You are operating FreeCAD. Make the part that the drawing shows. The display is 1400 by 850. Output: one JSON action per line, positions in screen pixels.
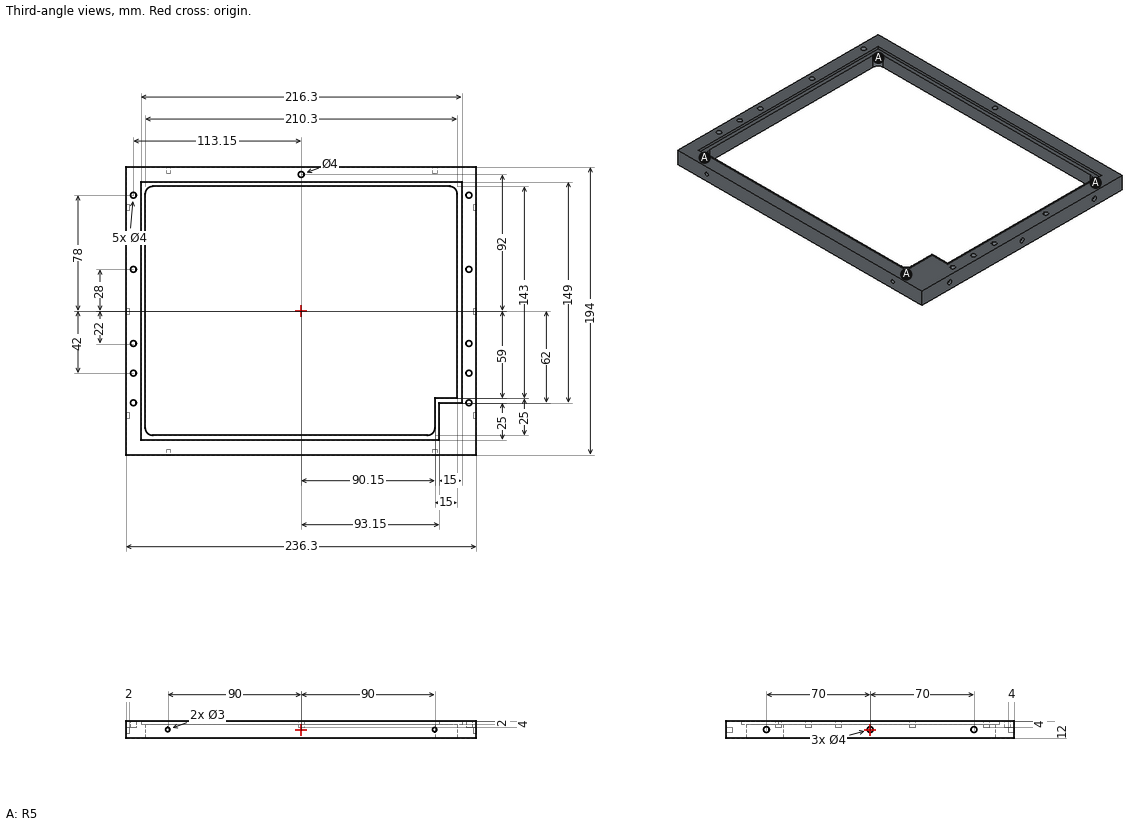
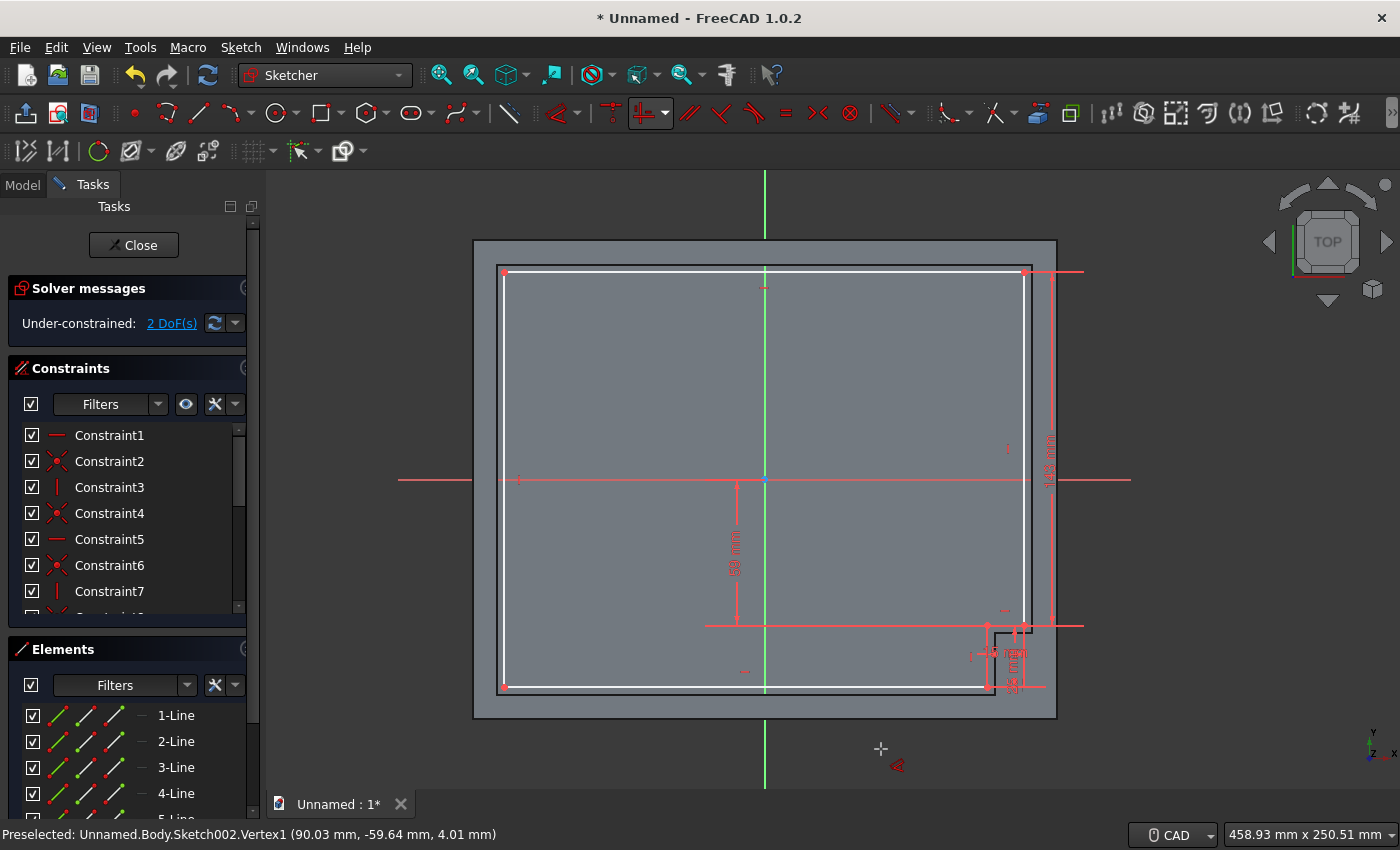
{"action": "left_click", "coordinate": [868, 272]}
{"action": "left_click", "coordinate": [645, 238]}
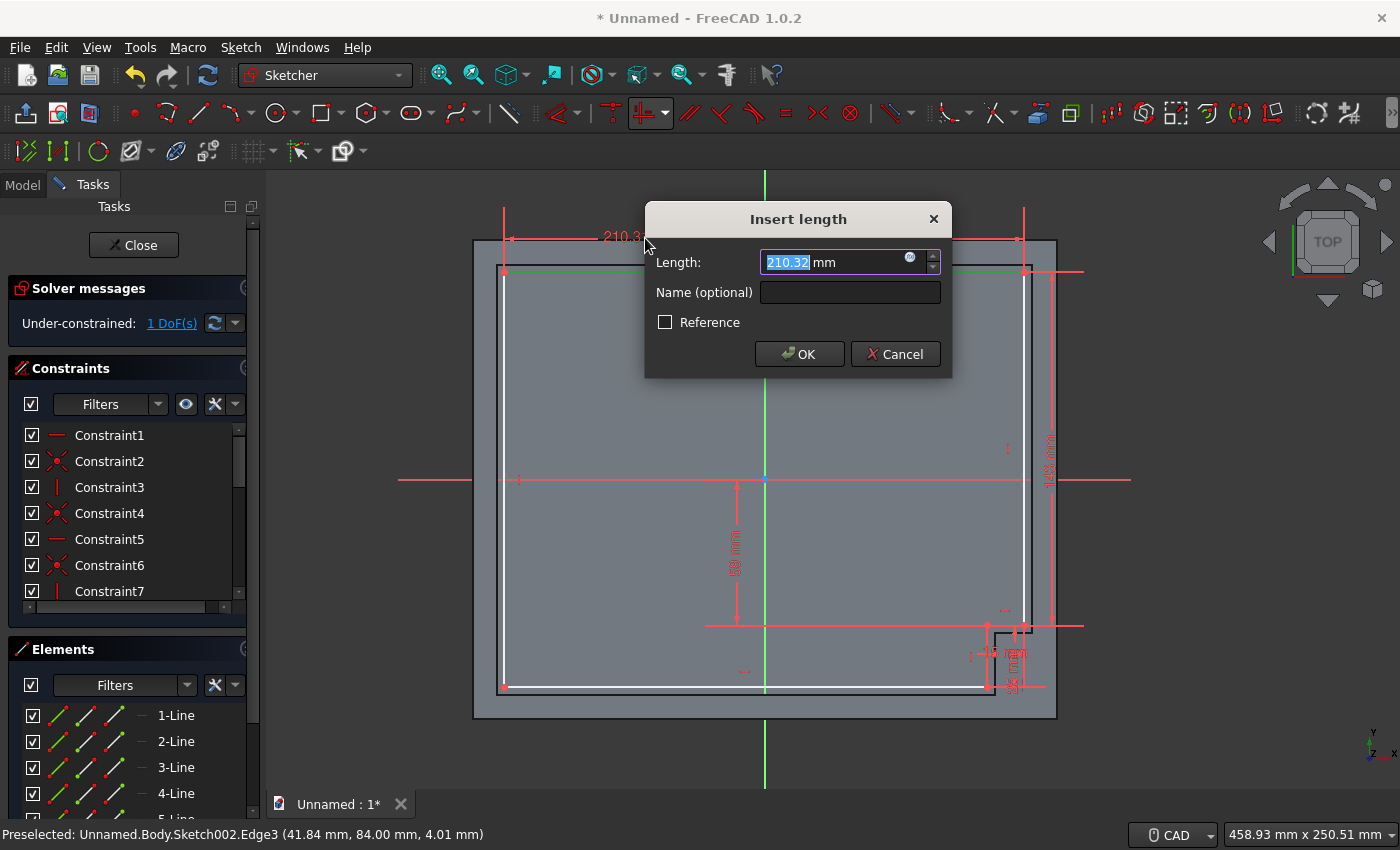
{"action": "type", "text": "210.3"}
{"action": "key", "text": "Return"}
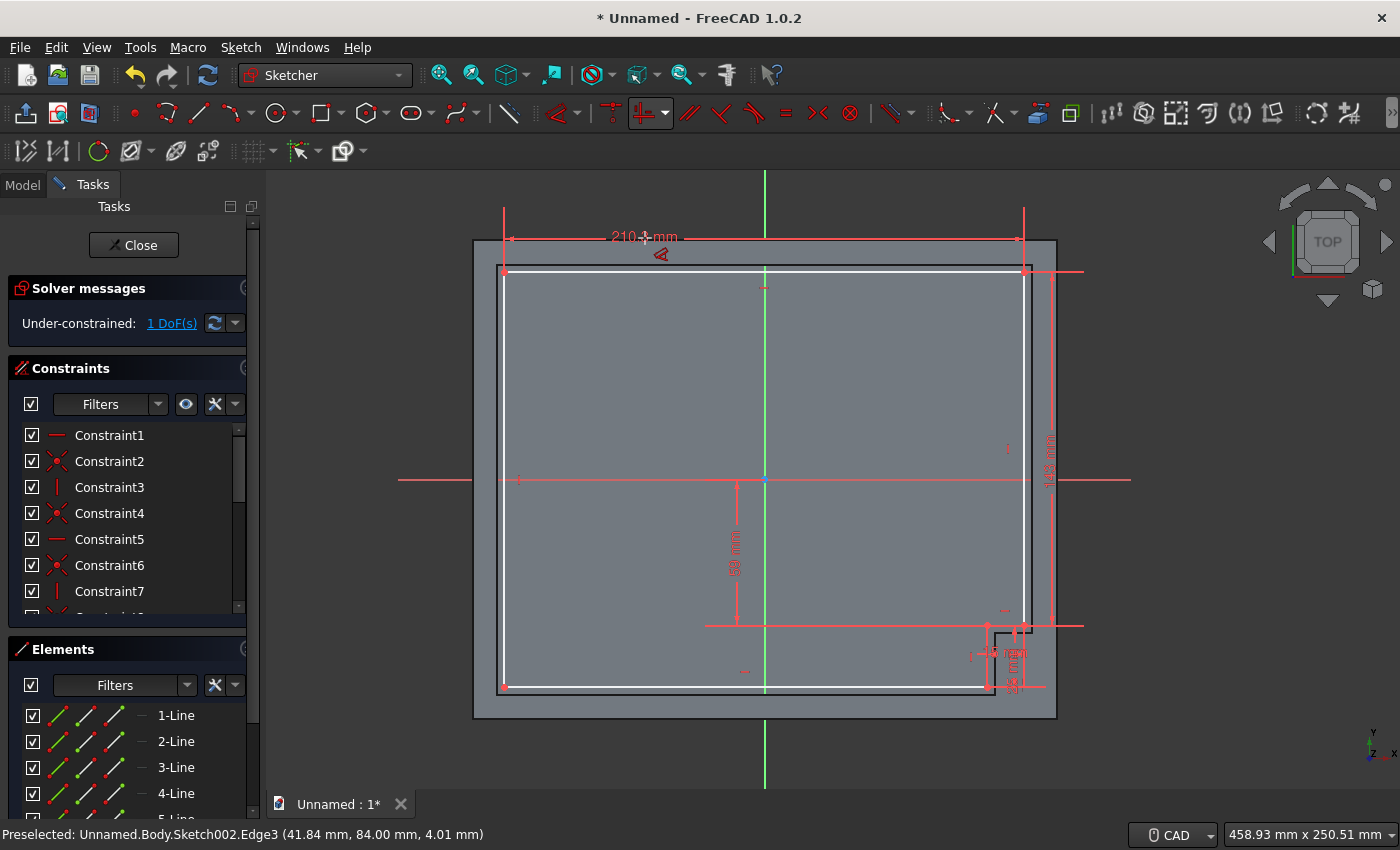
{"action": "left_click", "coordinate": [987, 626]}
{"action": "left_click", "coordinate": [876, 660]}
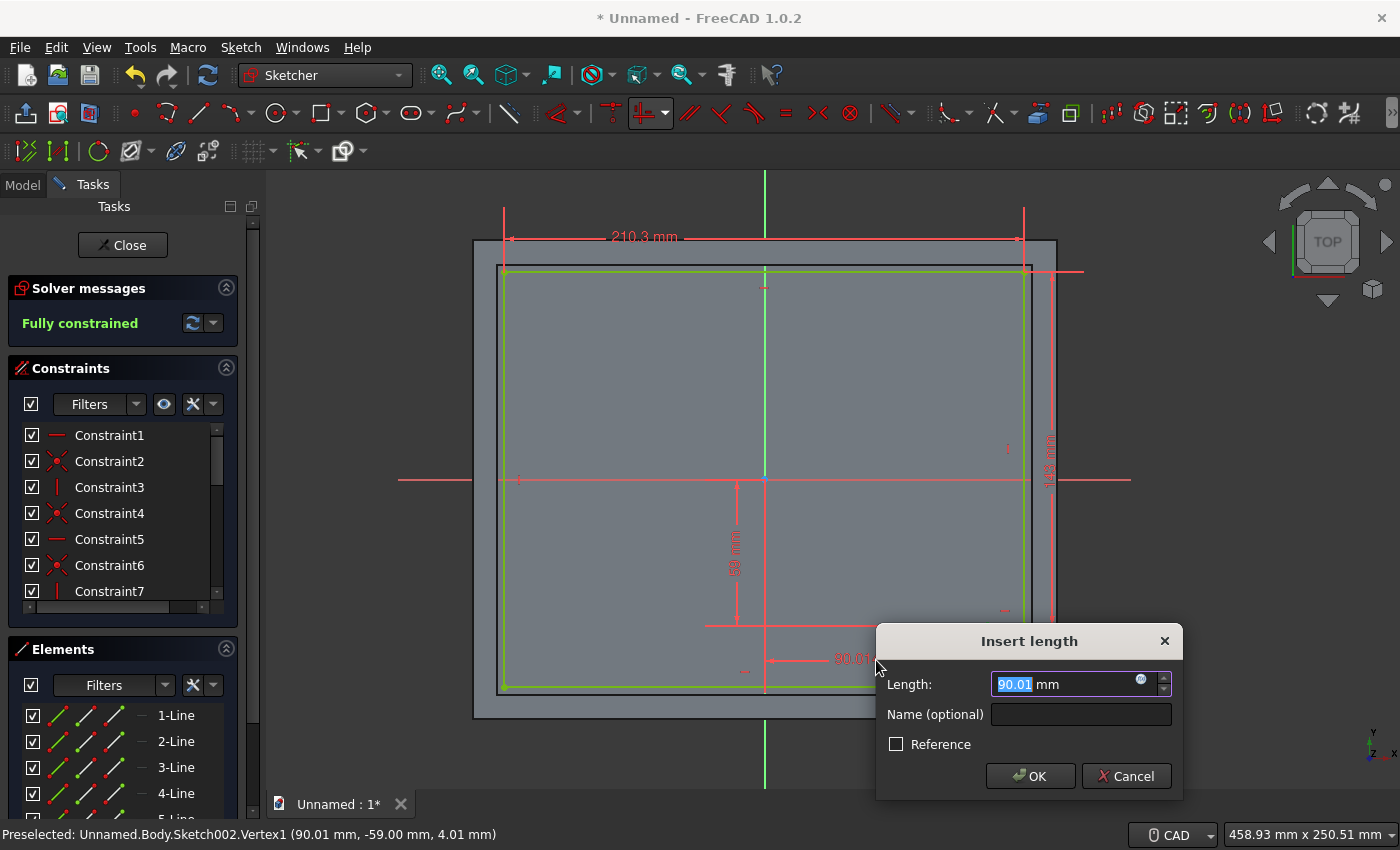
{"action": "type", "text": "90.15"}
{"action": "key", "text": "Return"}
{"action": "key", "text": "Escape"}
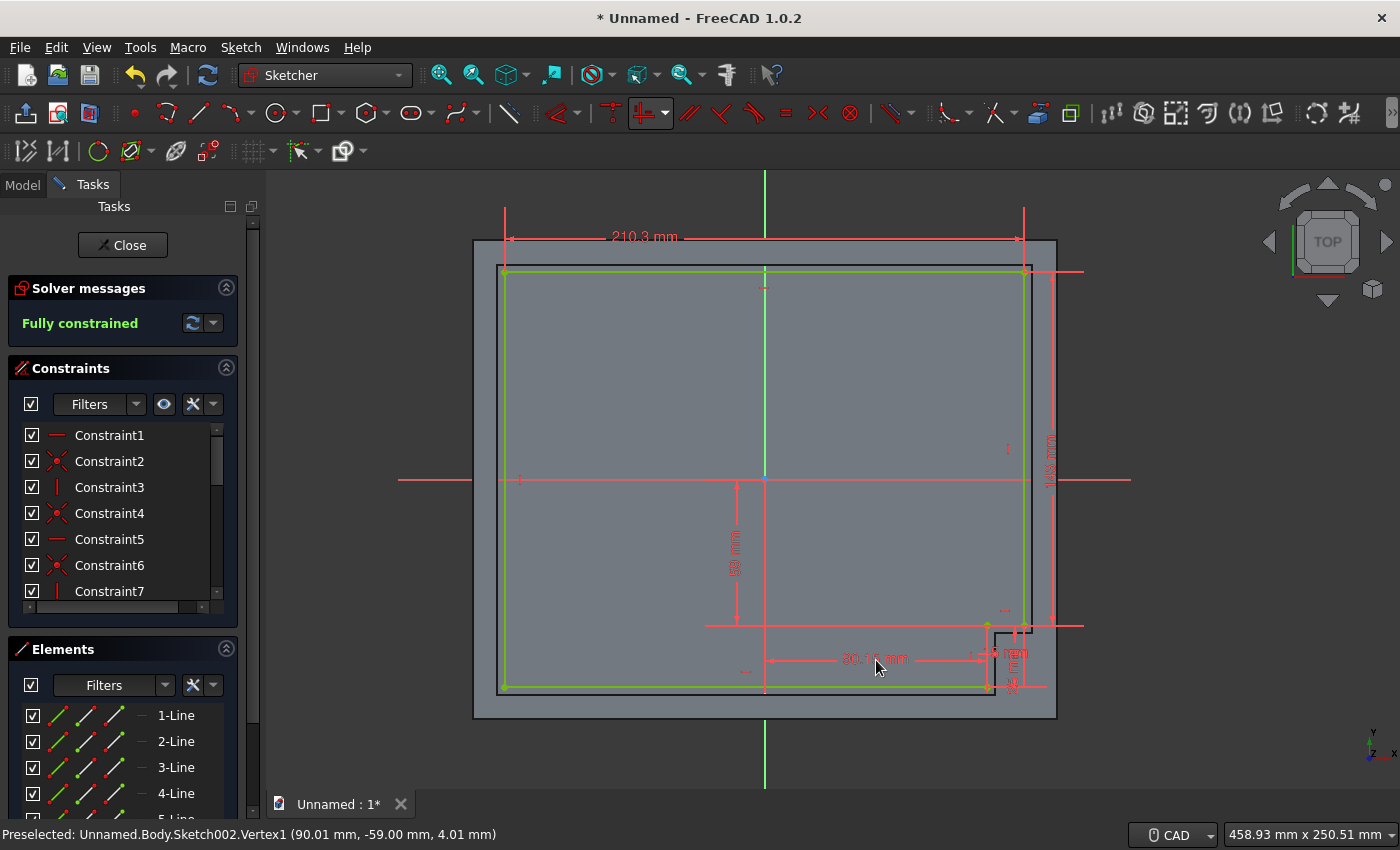
{"action": "left_click", "coordinate": [123, 245]}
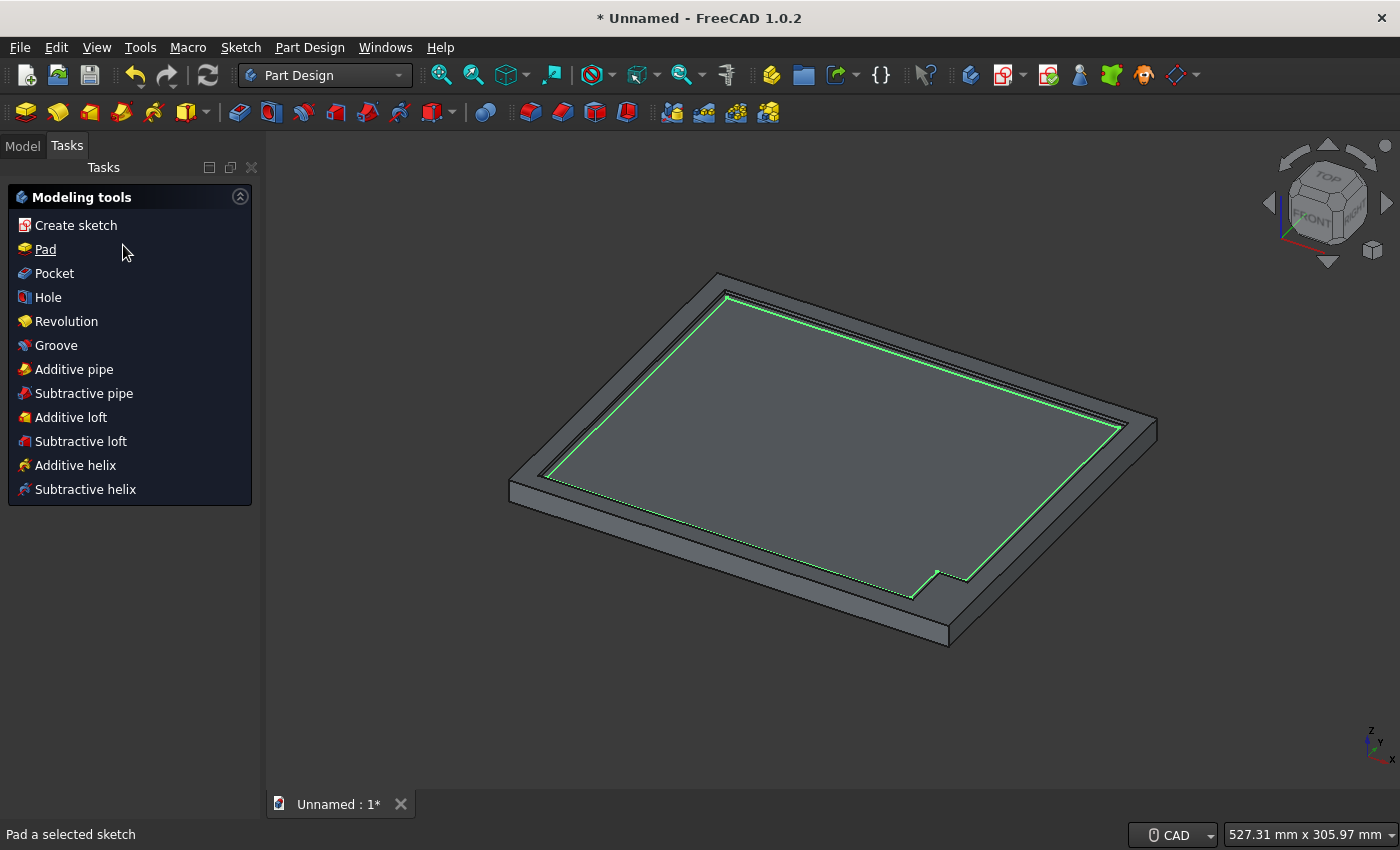
{"action": "left_click", "coordinate": [240, 112]}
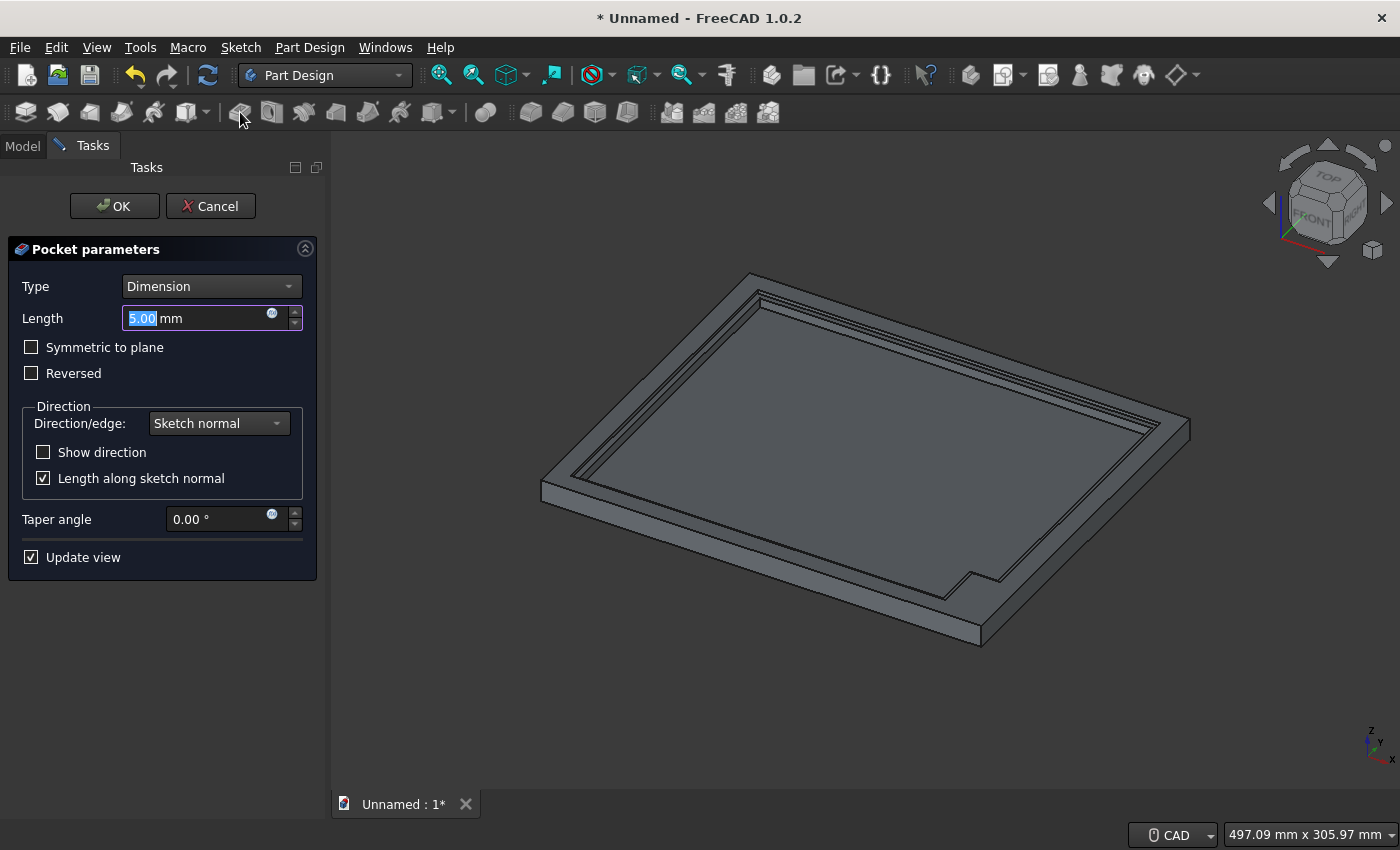
{"action": "left_click", "coordinate": [212, 286]}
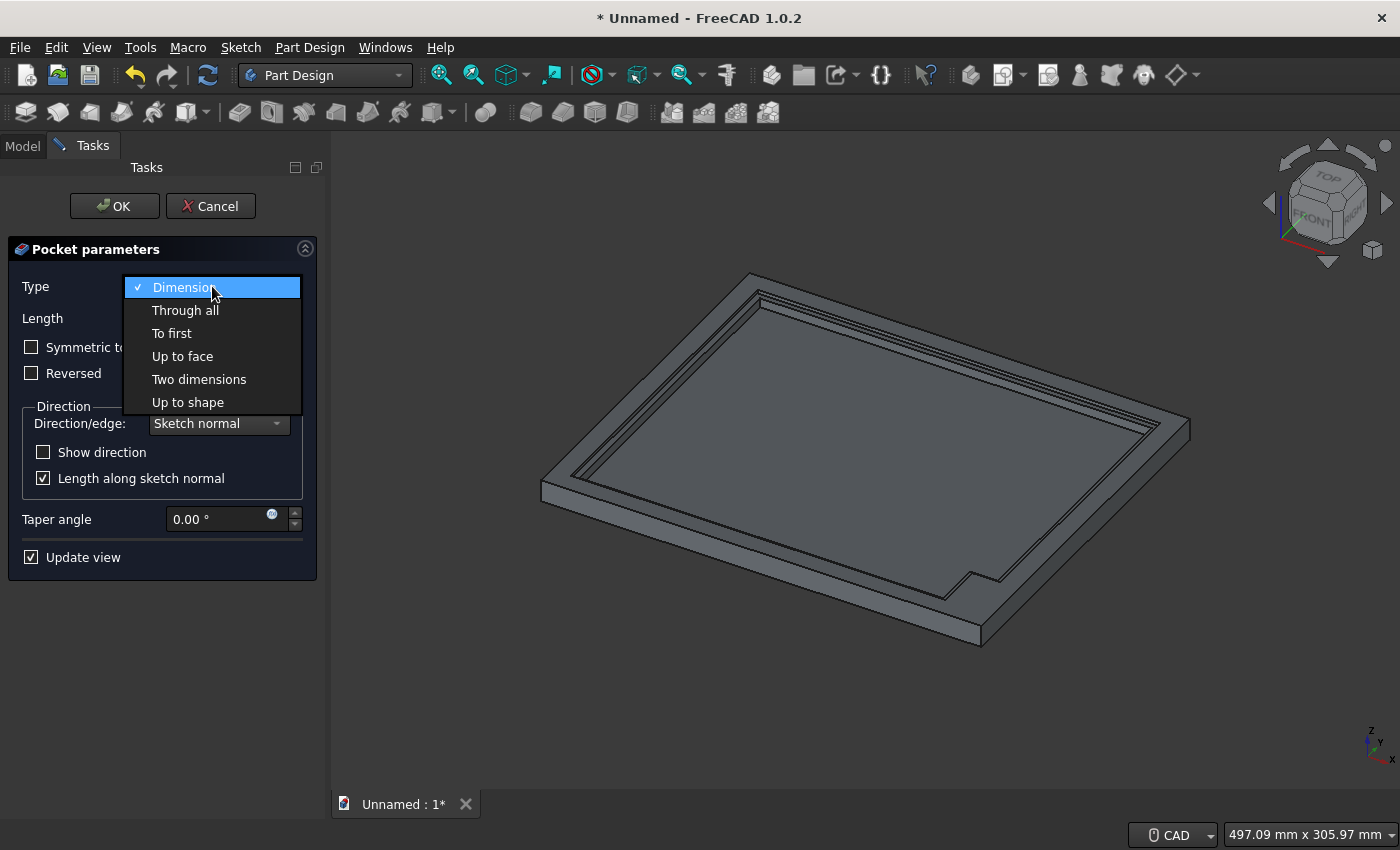
{"action": "left_click", "coordinate": [212, 310]}